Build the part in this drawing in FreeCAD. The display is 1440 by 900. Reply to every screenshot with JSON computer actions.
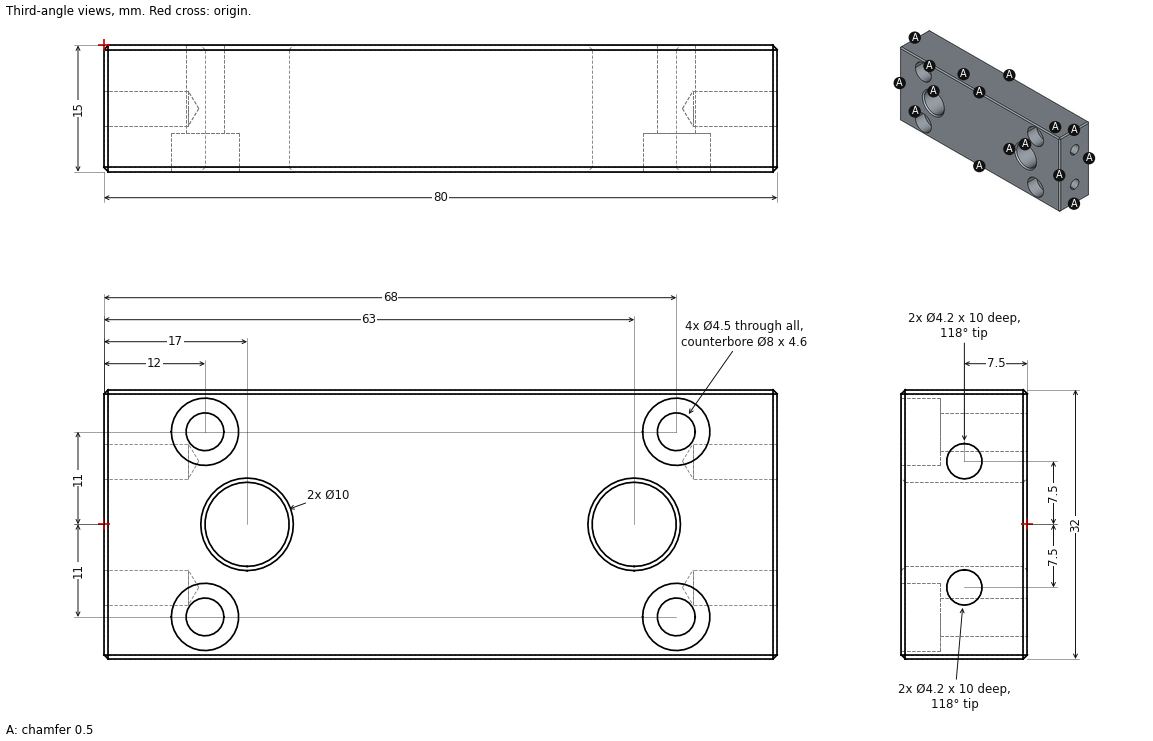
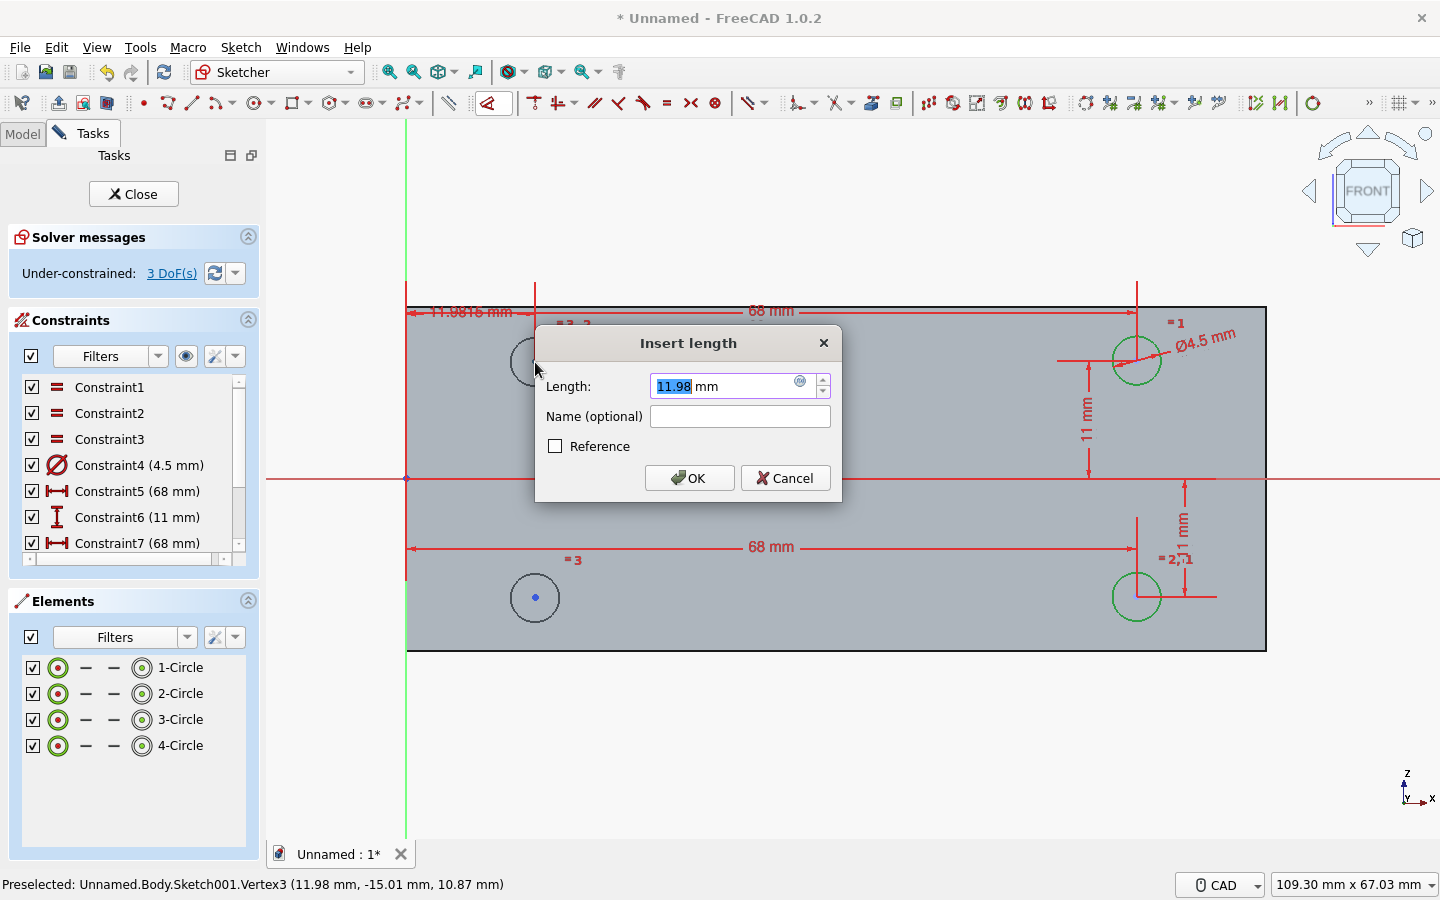
{"action": "type", "text": "12"}
{"action": "key", "text": "Return"}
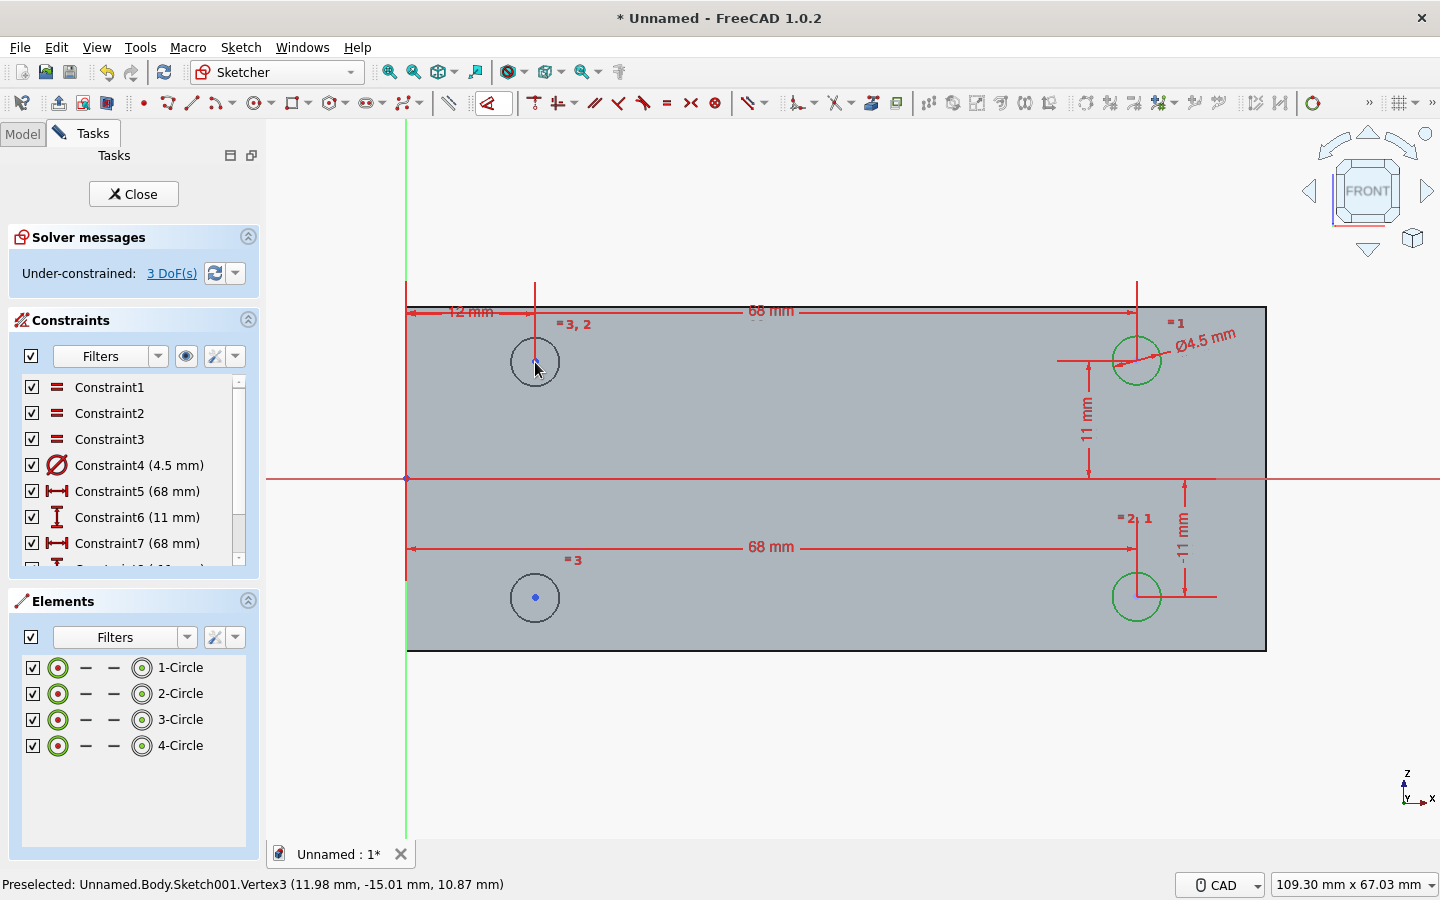
{"action": "left_click", "coordinate": [535, 362]}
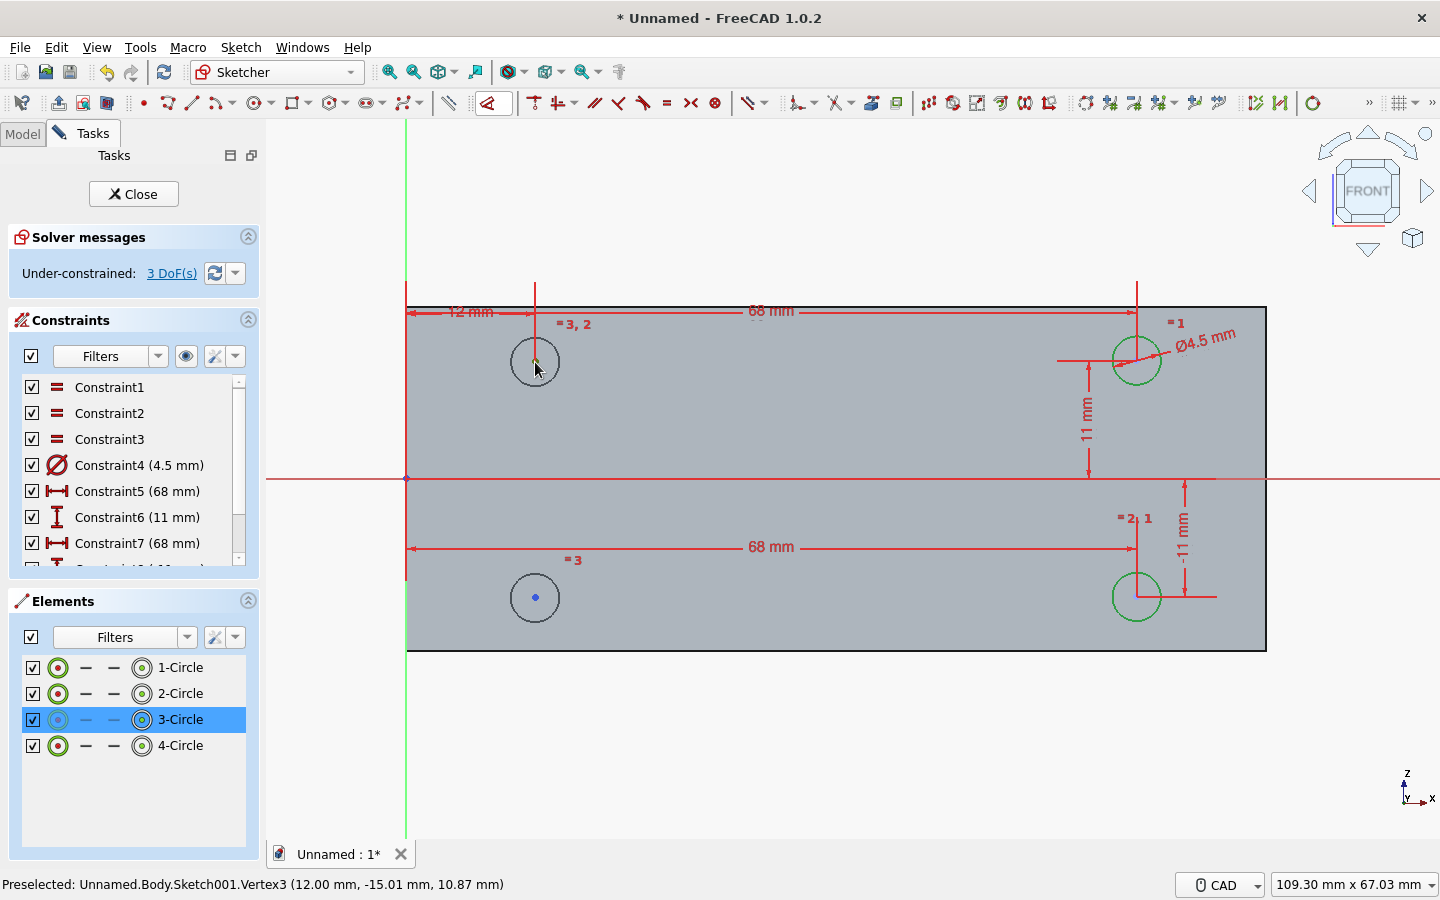
{"action": "key", "text": "i"}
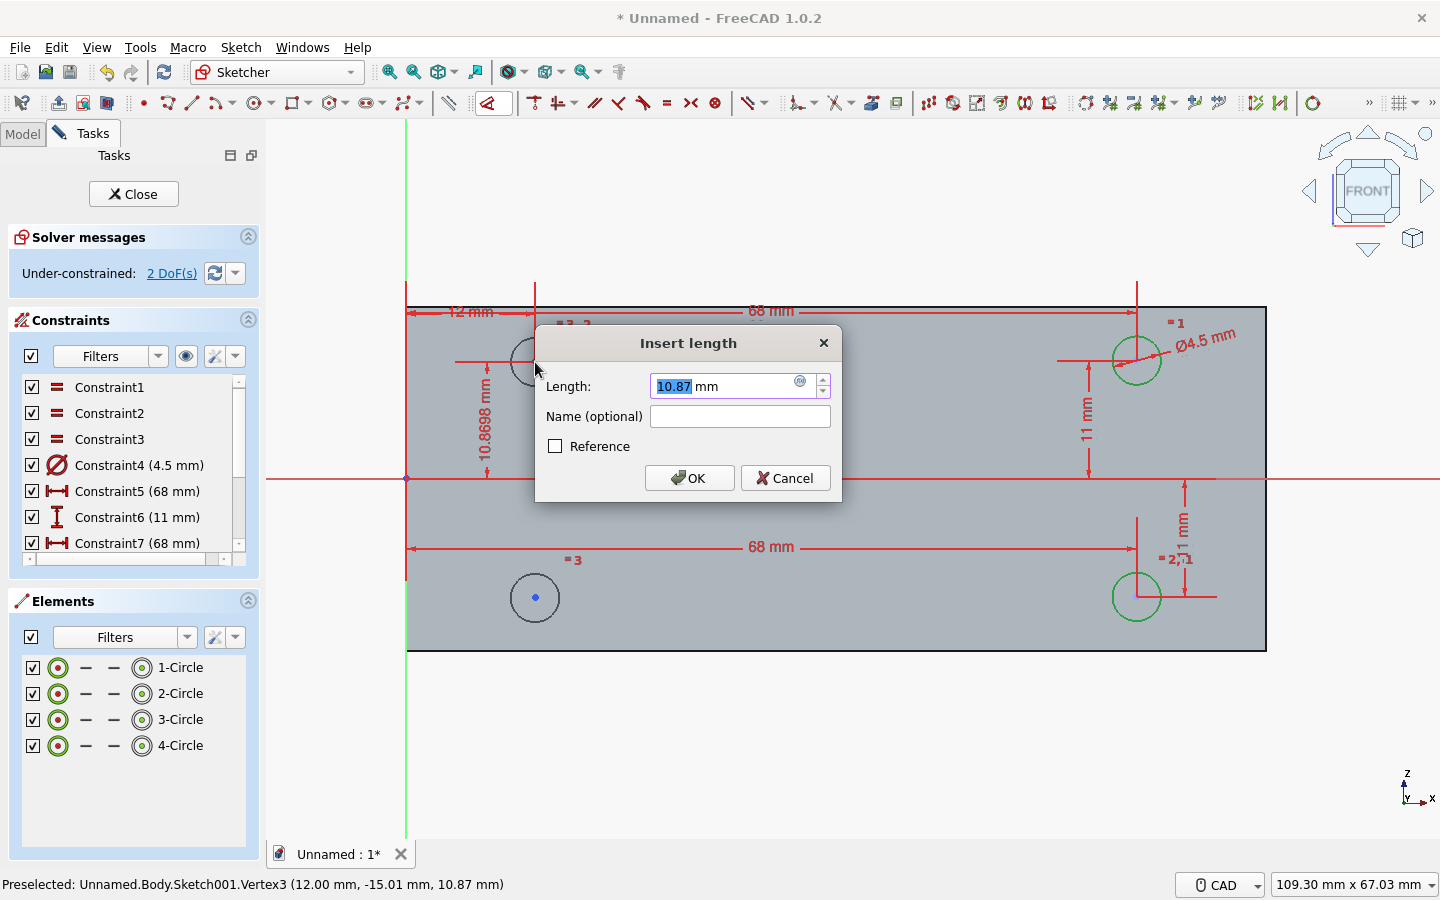
{"action": "type", "text": "11"}
{"action": "key", "text": "Return"}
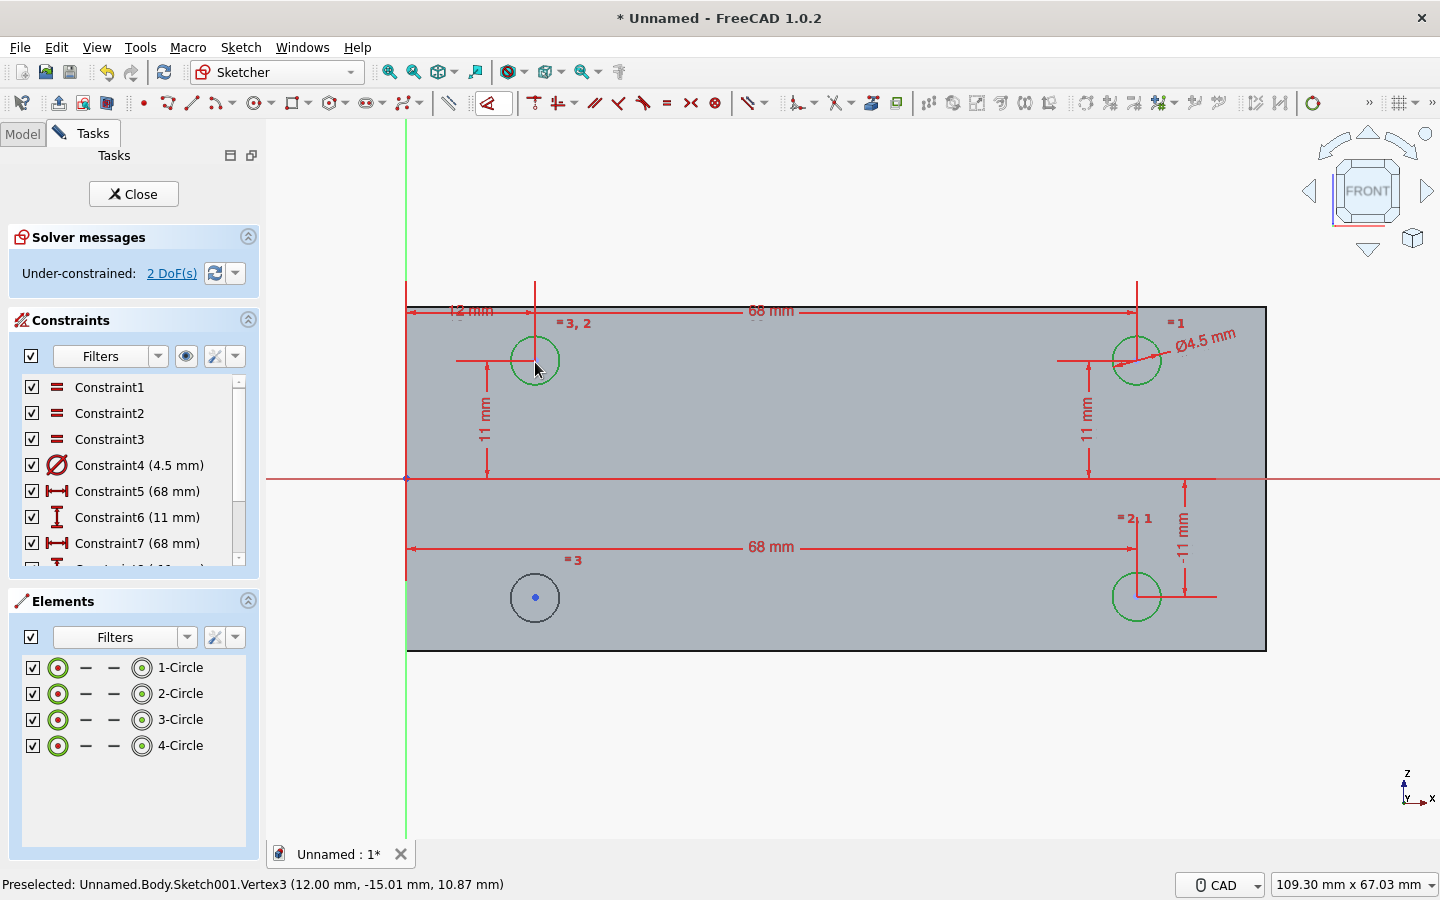
{"action": "left_click", "coordinate": [535, 598]}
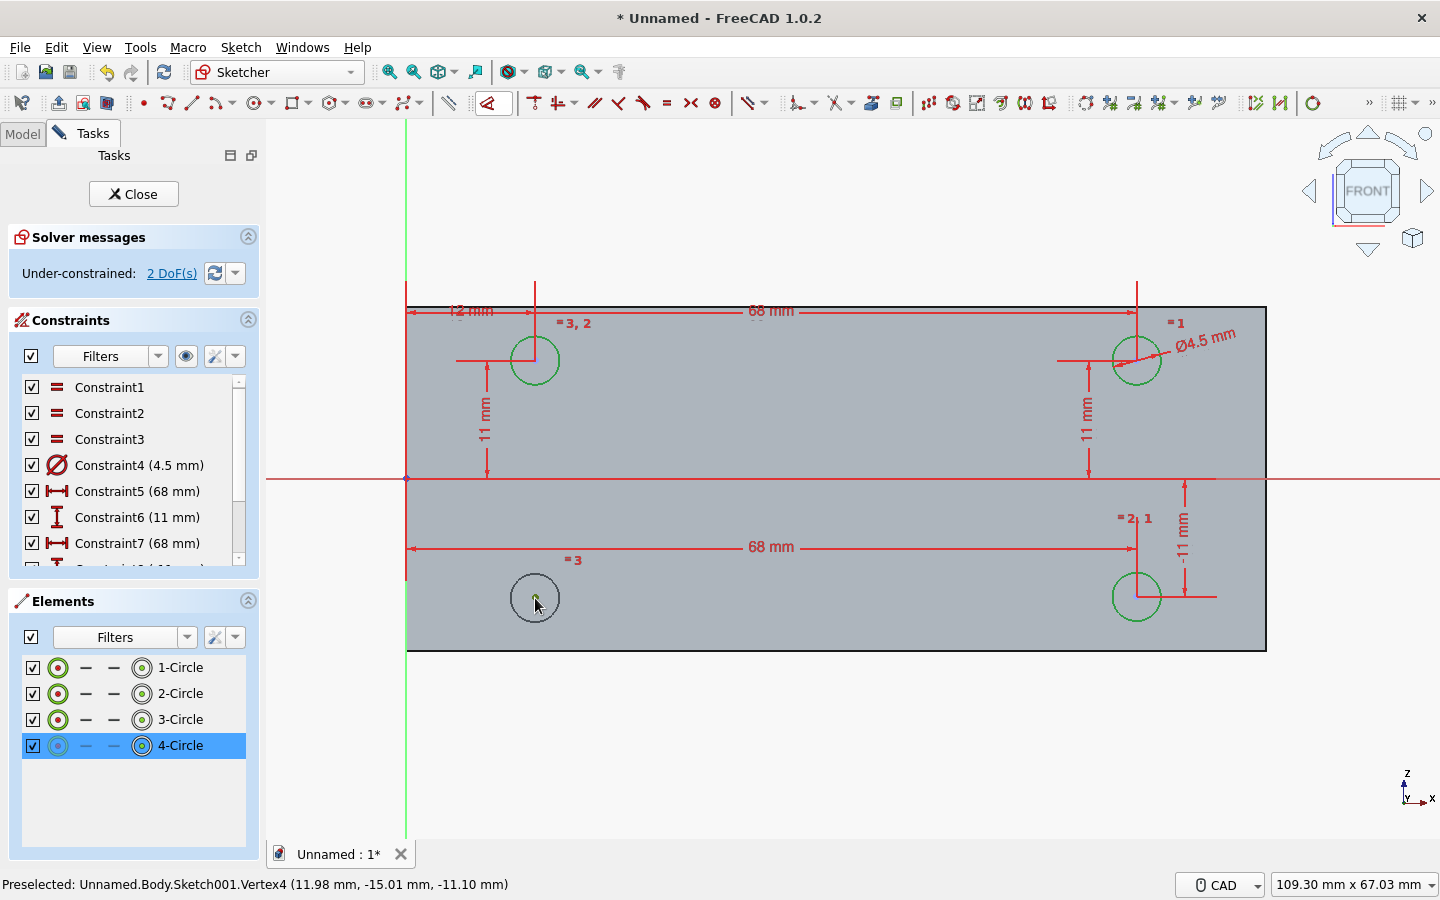
{"action": "left_click", "coordinate": [506, 104]}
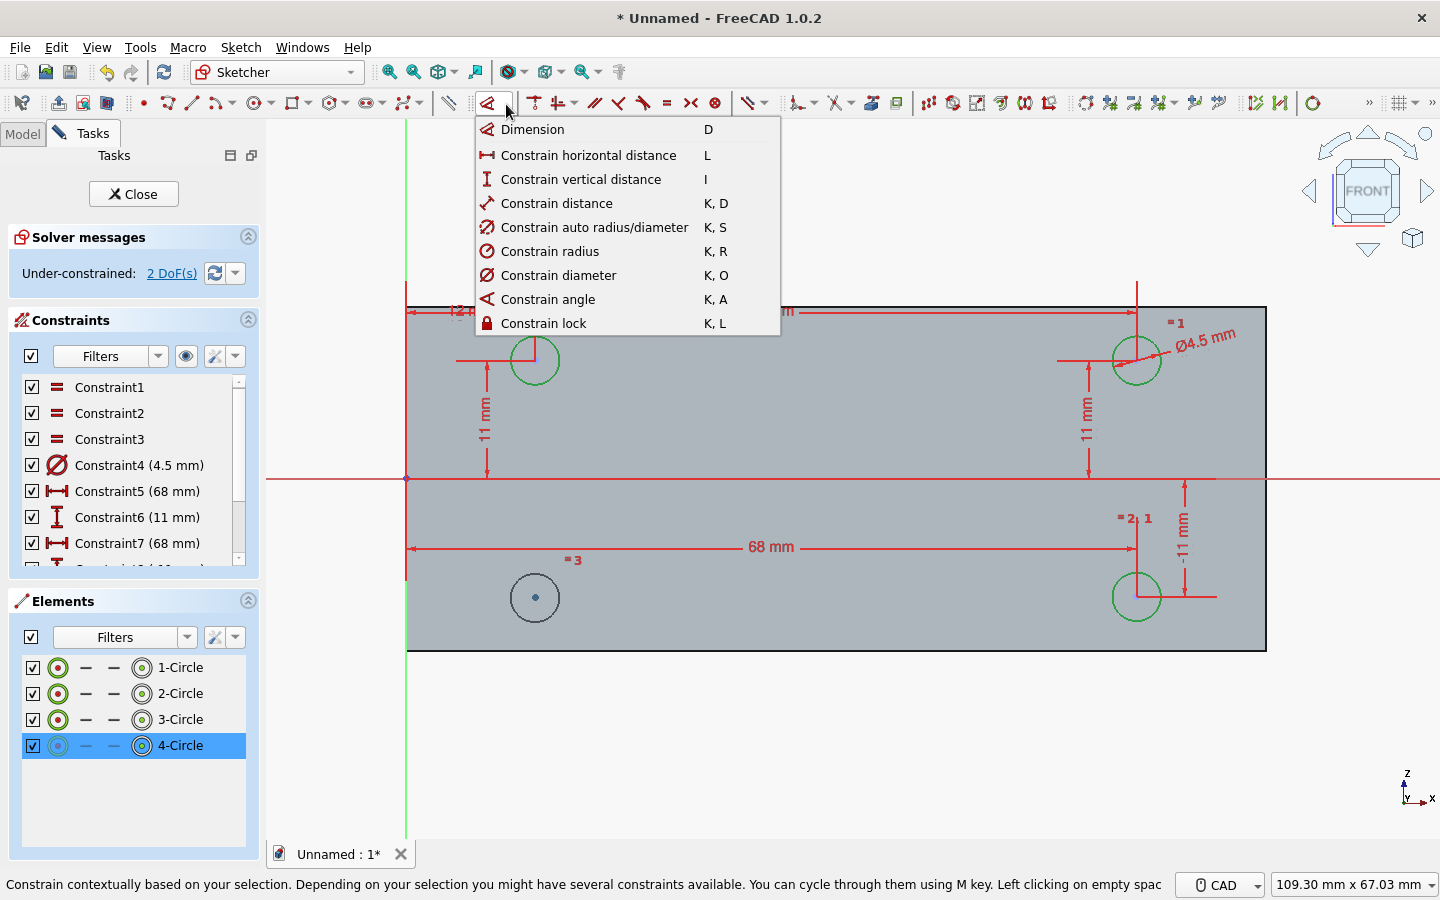
{"action": "left_click", "coordinate": [628, 155]}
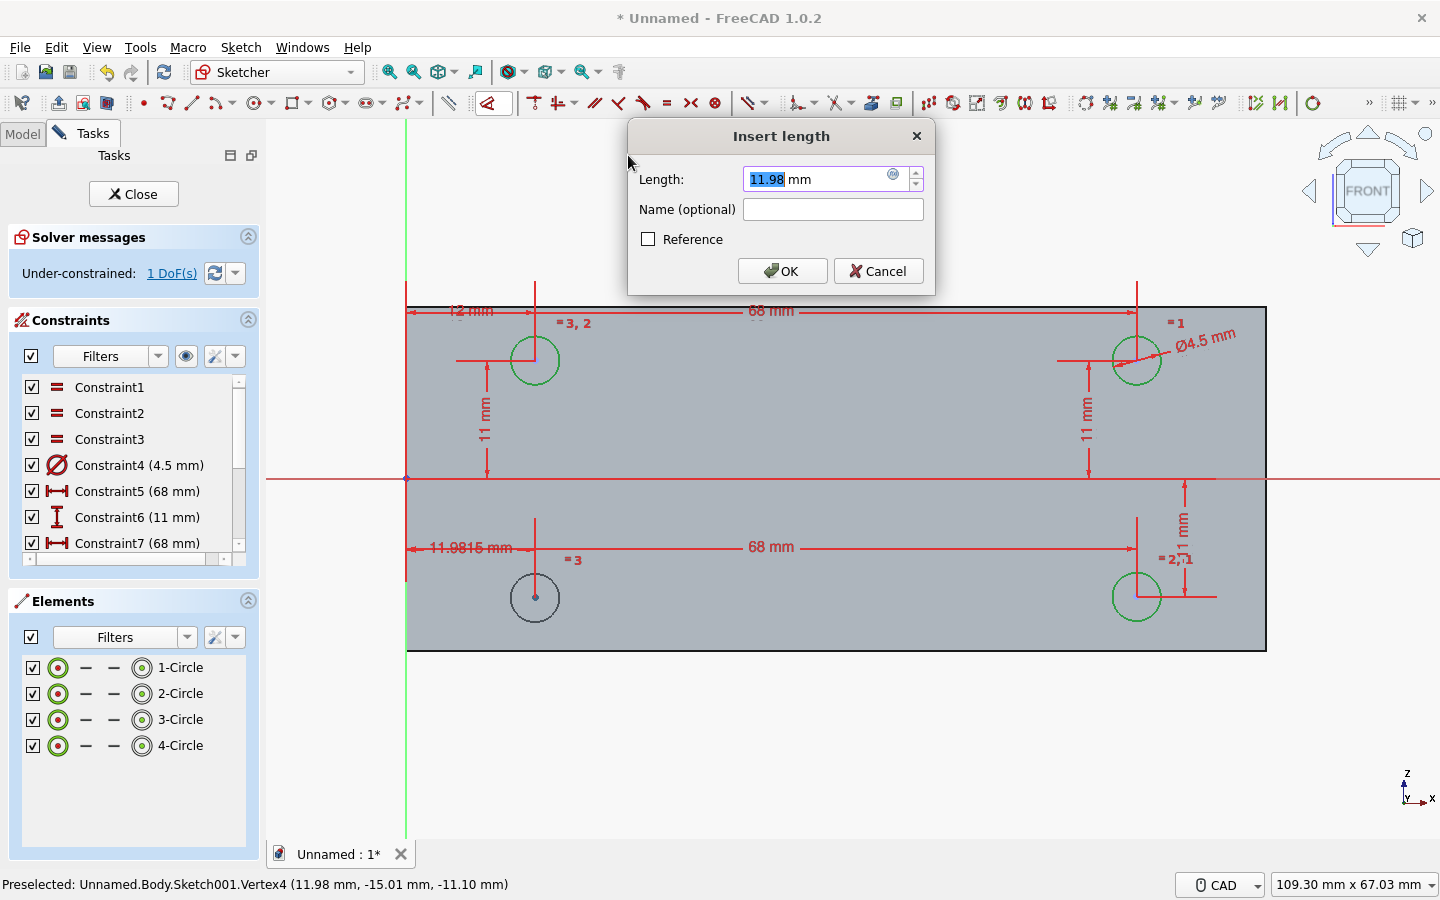
{"action": "type", "text": "12"}
{"action": "key", "text": "Return"}